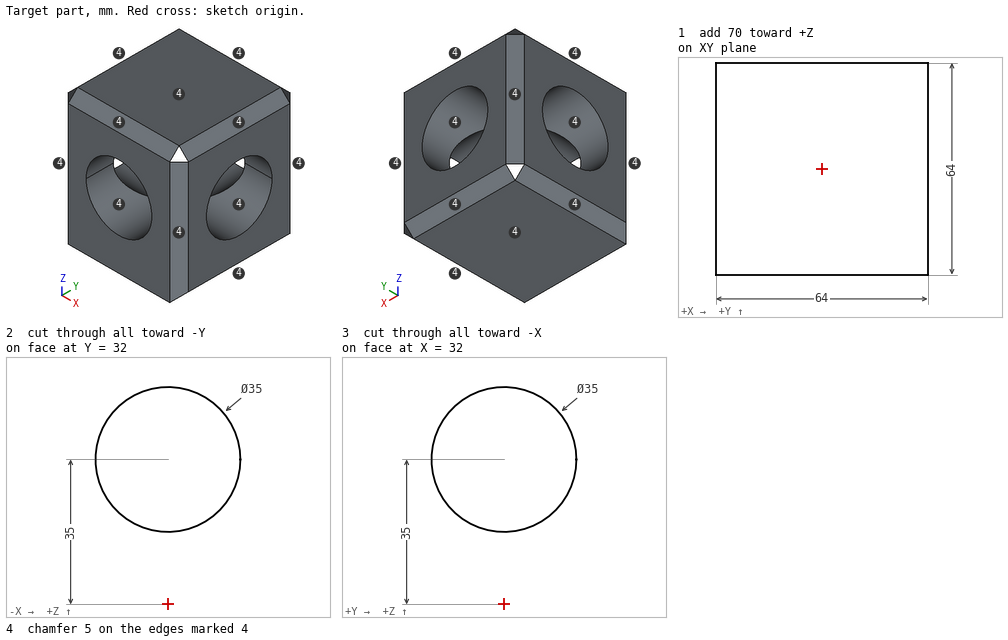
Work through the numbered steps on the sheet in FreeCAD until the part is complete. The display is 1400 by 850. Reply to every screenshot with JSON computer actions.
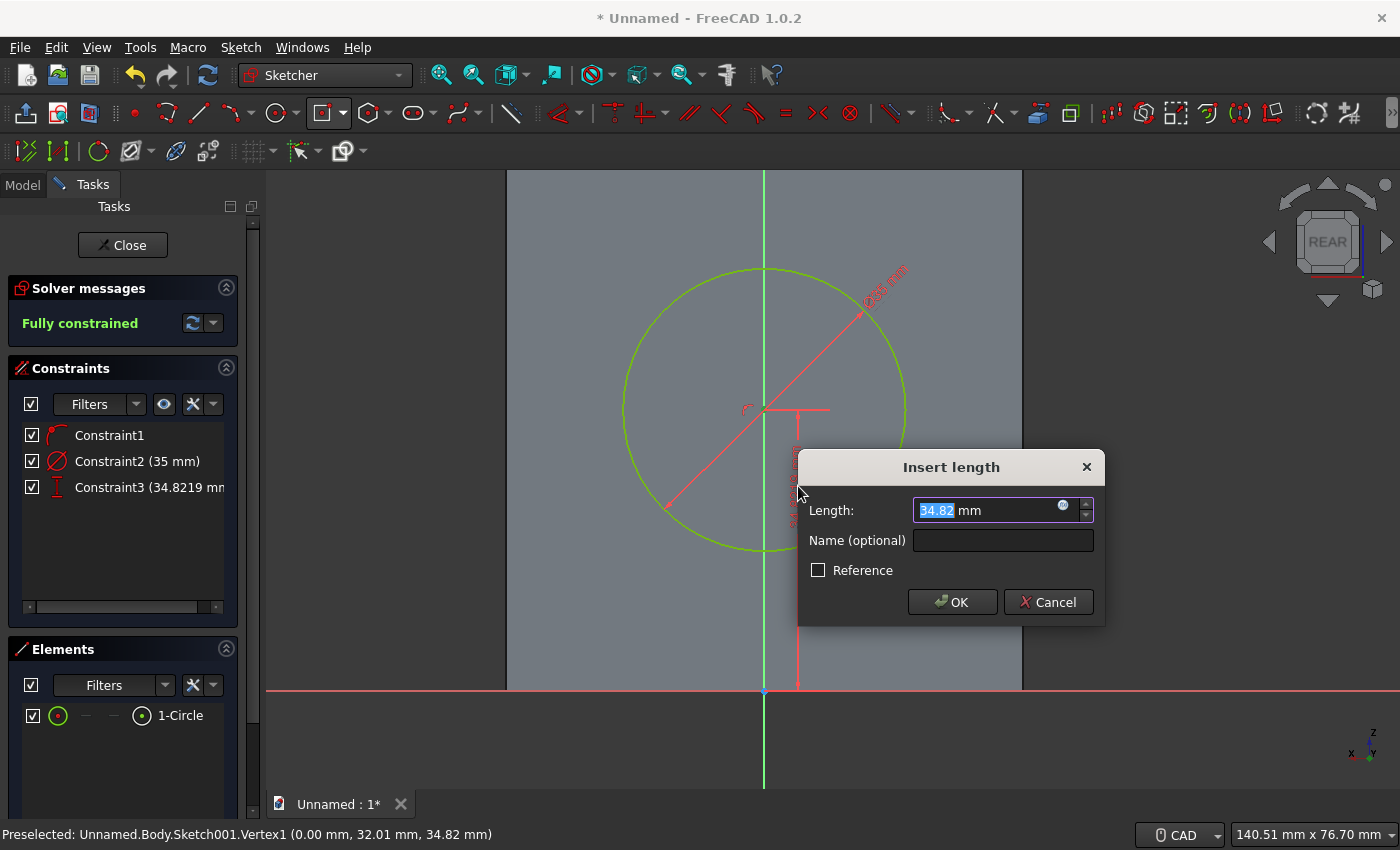
{"action": "type", "text": "35"}
{"action": "key", "text": "Return"}
{"action": "key", "text": "Escape"}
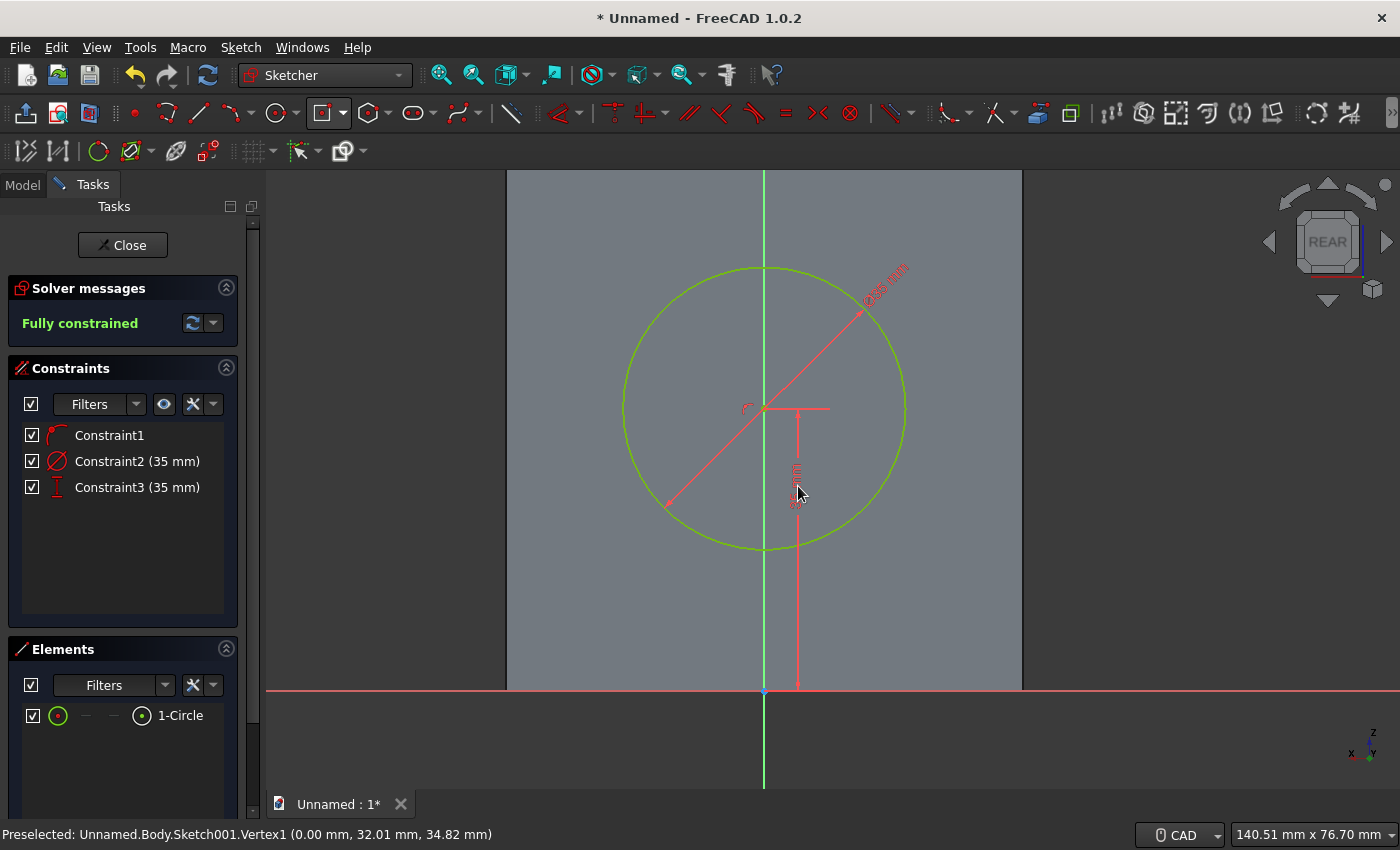
{"action": "left_click", "coordinate": [123, 245]}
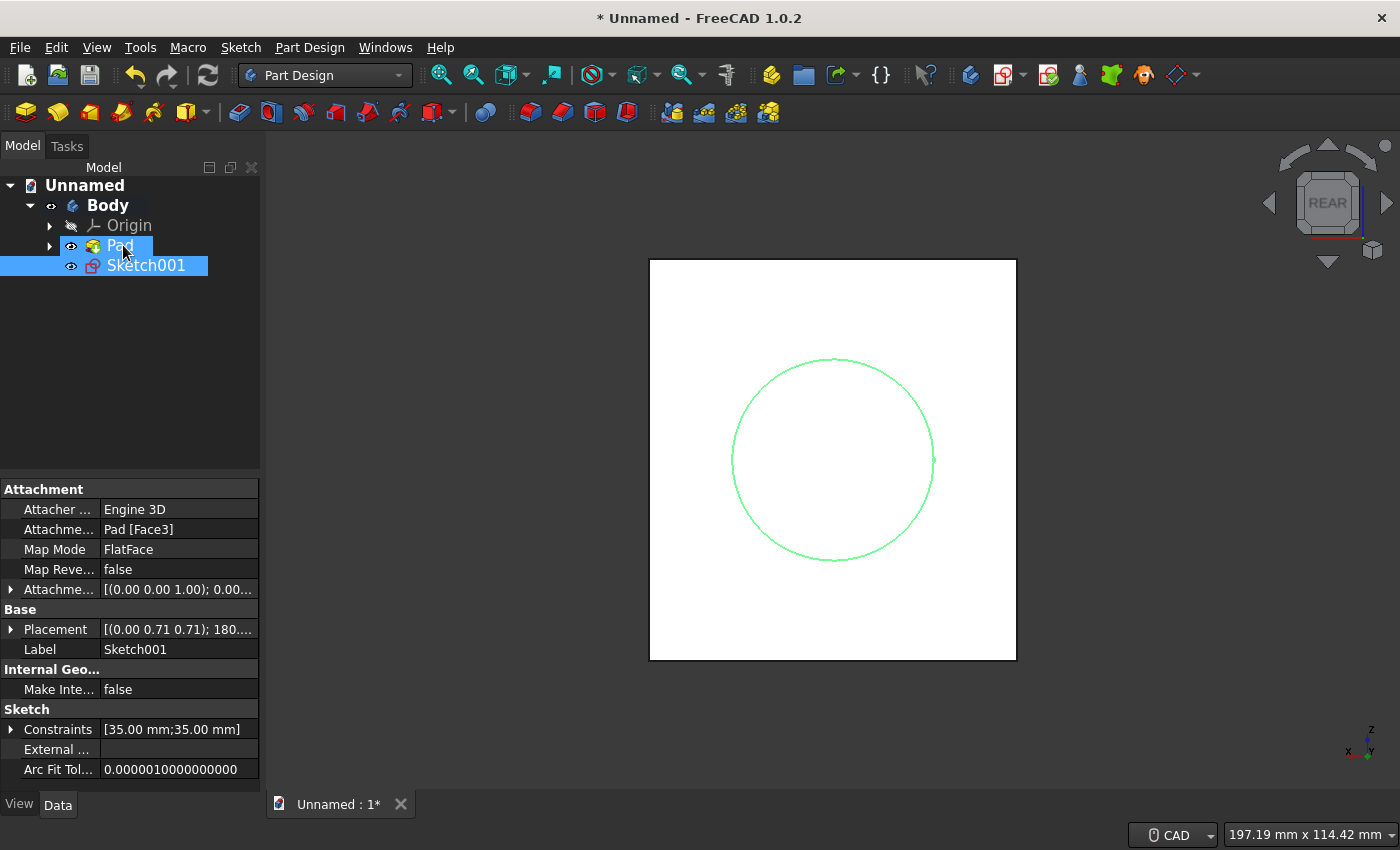
{"action": "left_click", "coordinate": [240, 112]}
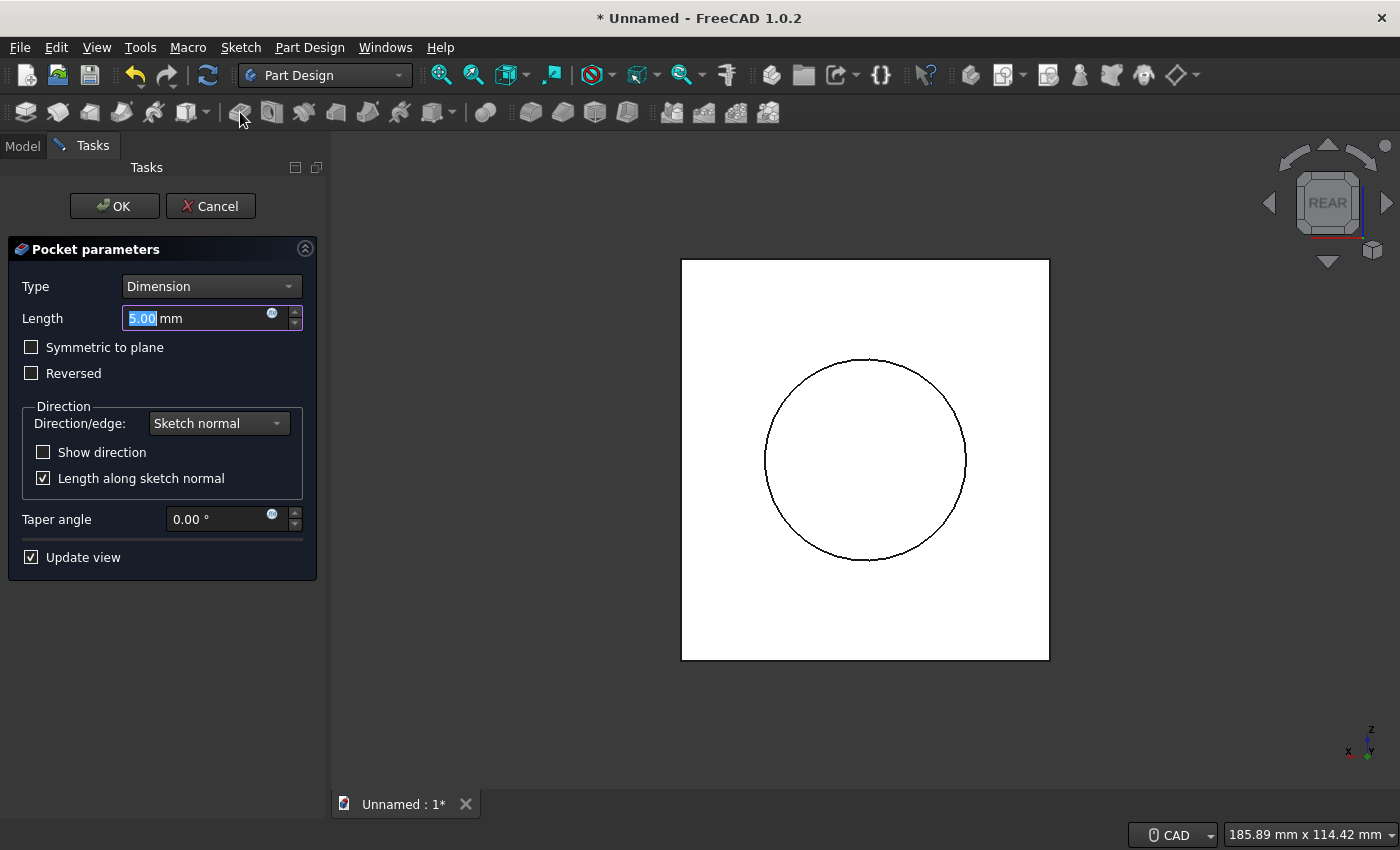
{"action": "left_click", "coordinate": [212, 286]}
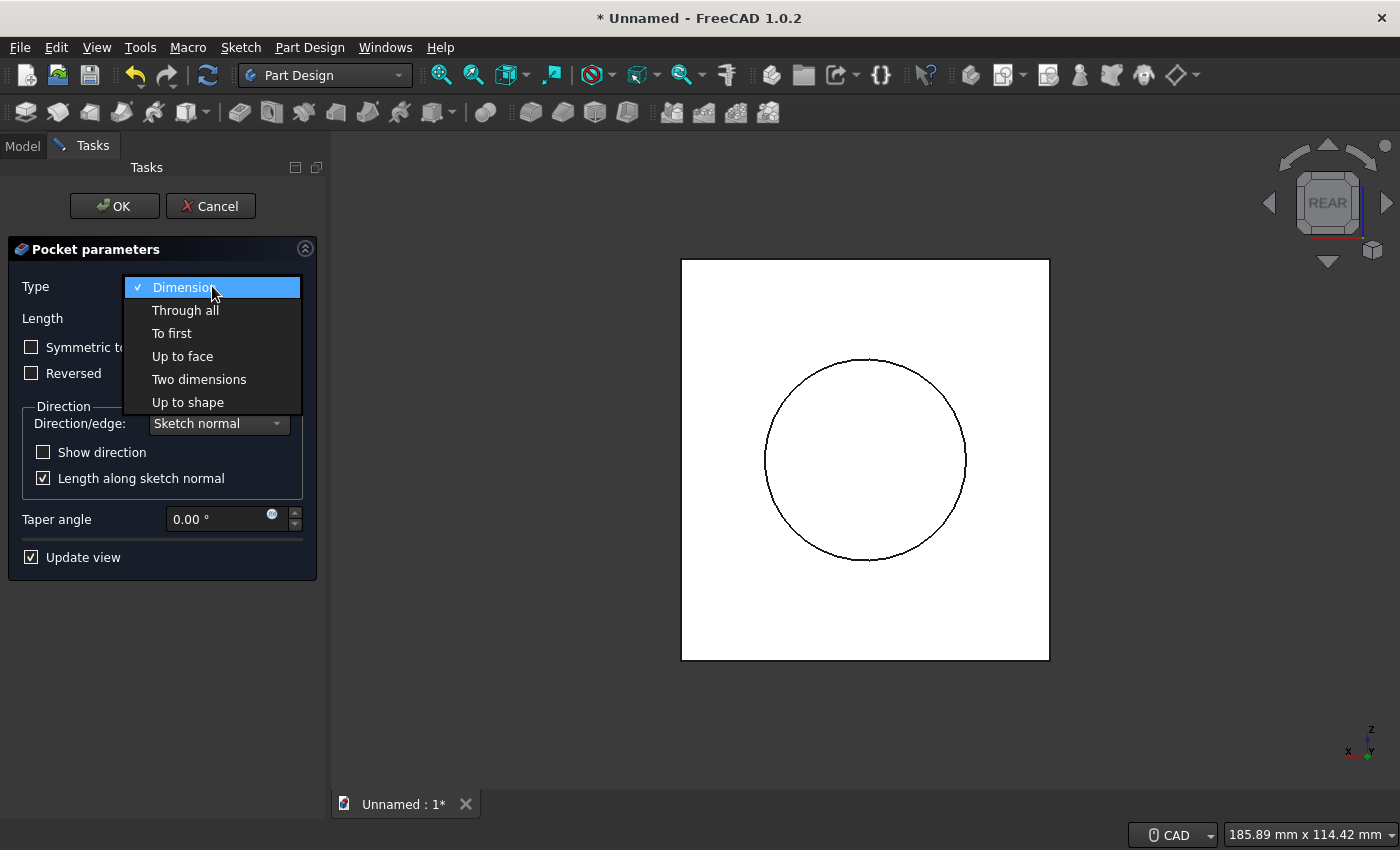
{"action": "left_click", "coordinate": [212, 310]}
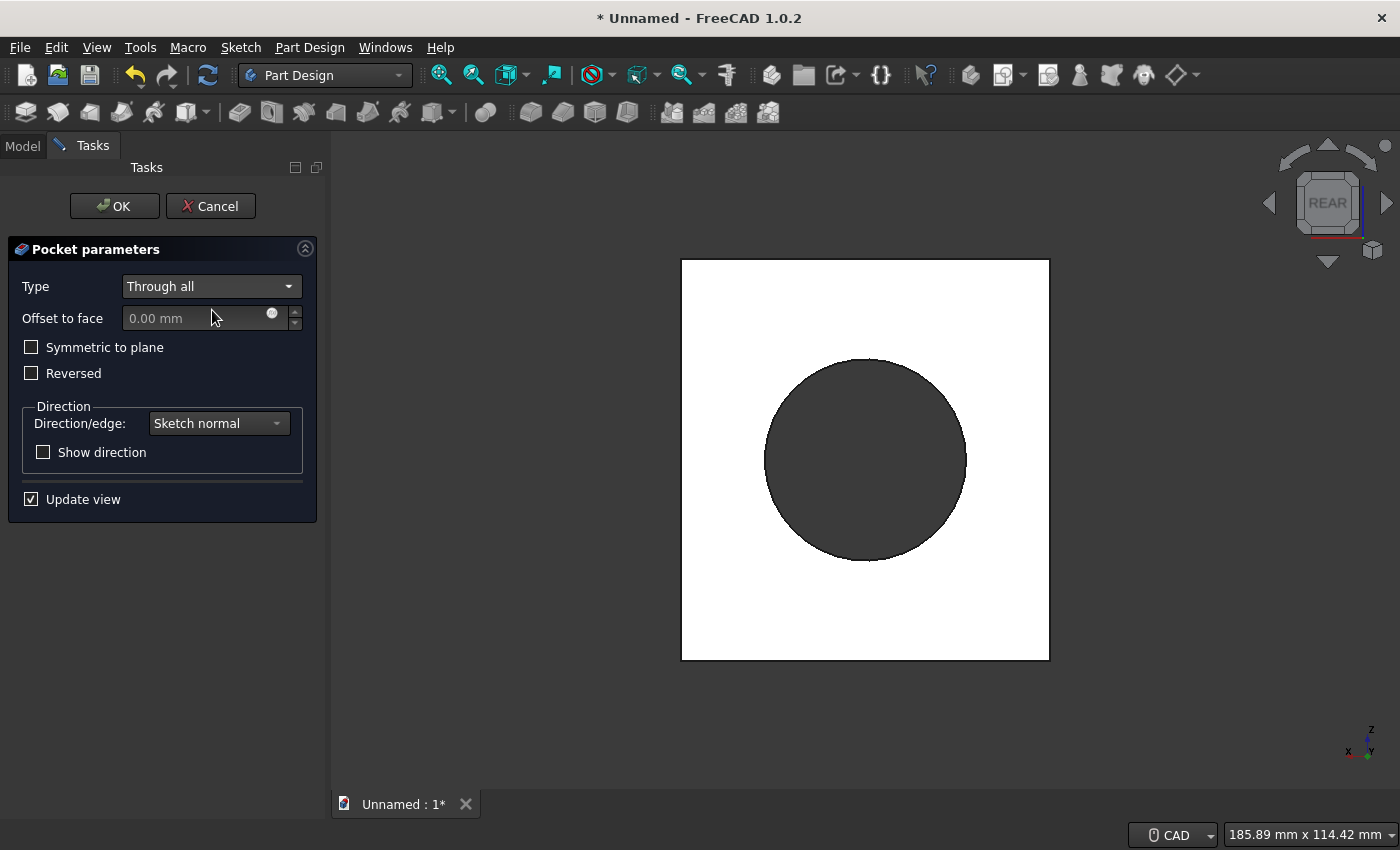
{"action": "left_click", "coordinate": [115, 206]}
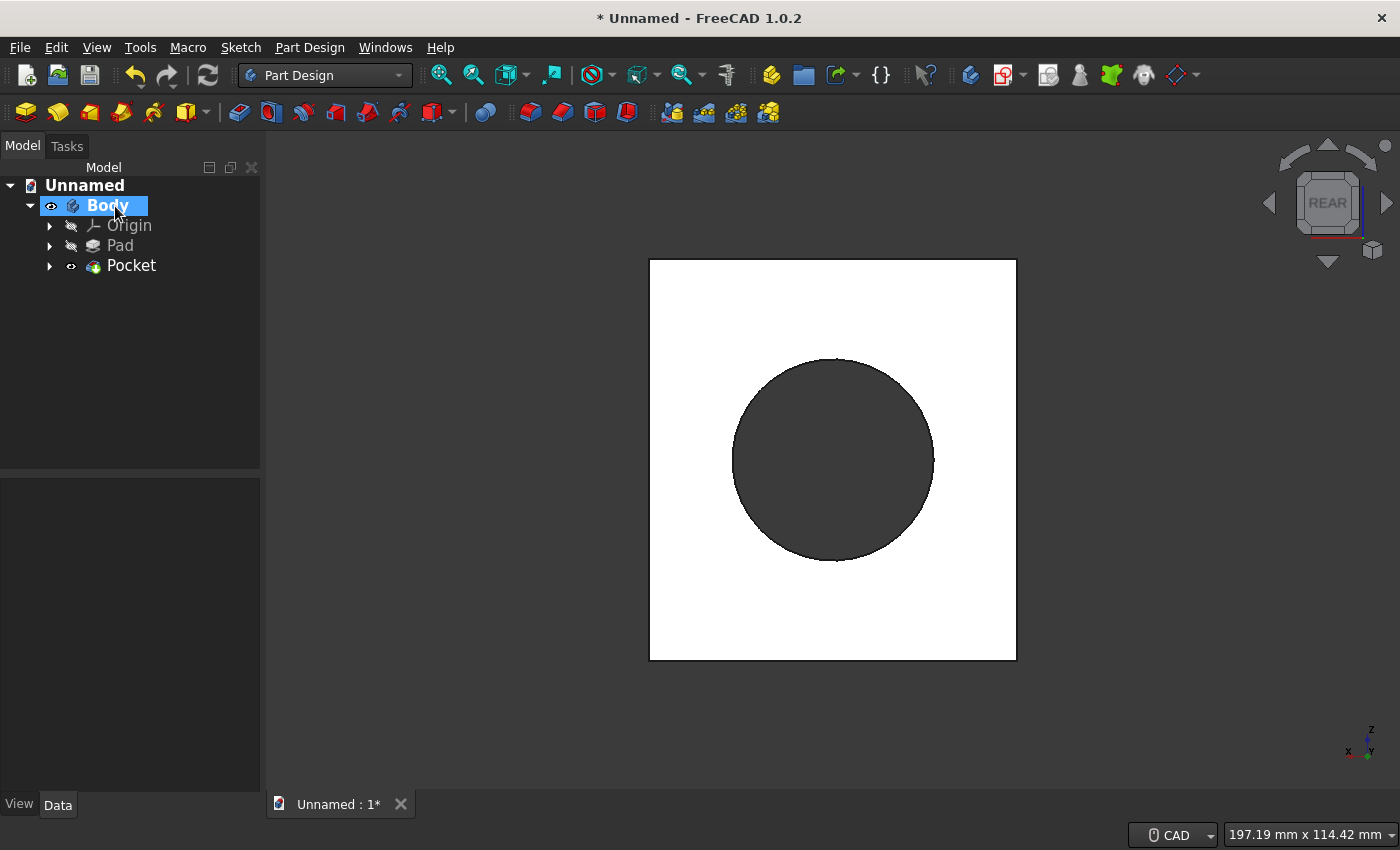
{"action": "key", "text": "0"}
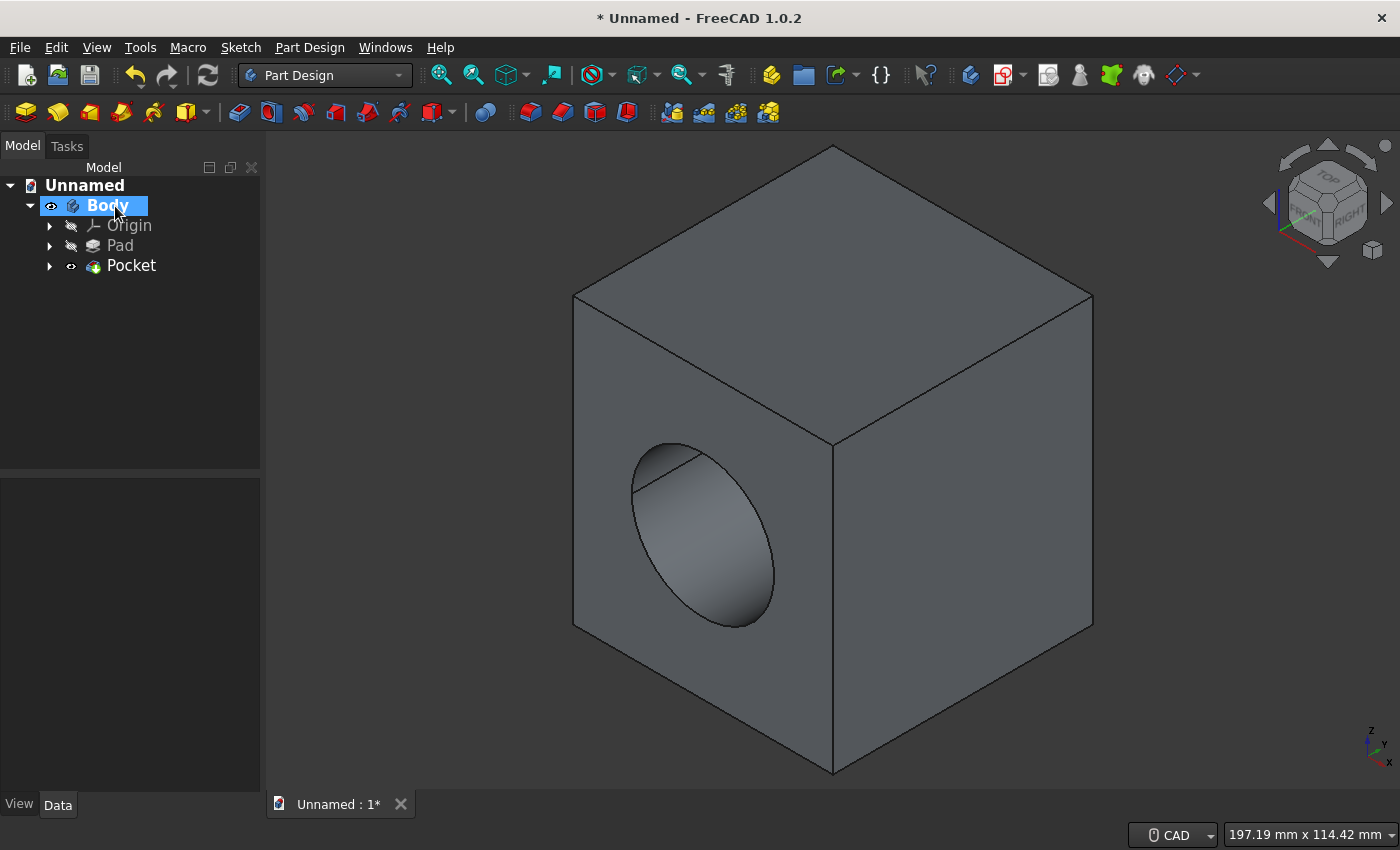
{"action": "left_click", "coordinate": [963, 534]}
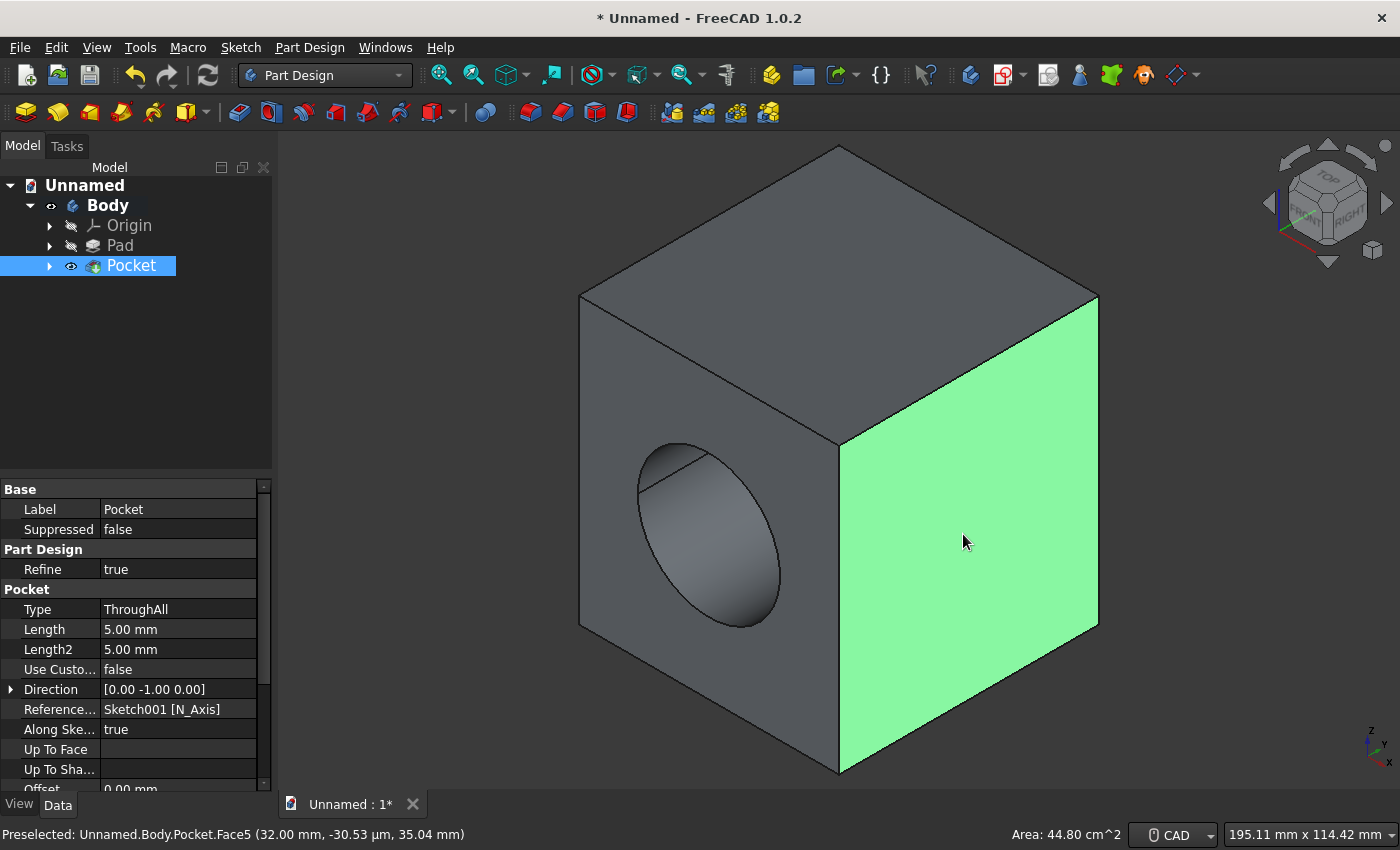
{"action": "left_click", "coordinate": [1004, 76]}